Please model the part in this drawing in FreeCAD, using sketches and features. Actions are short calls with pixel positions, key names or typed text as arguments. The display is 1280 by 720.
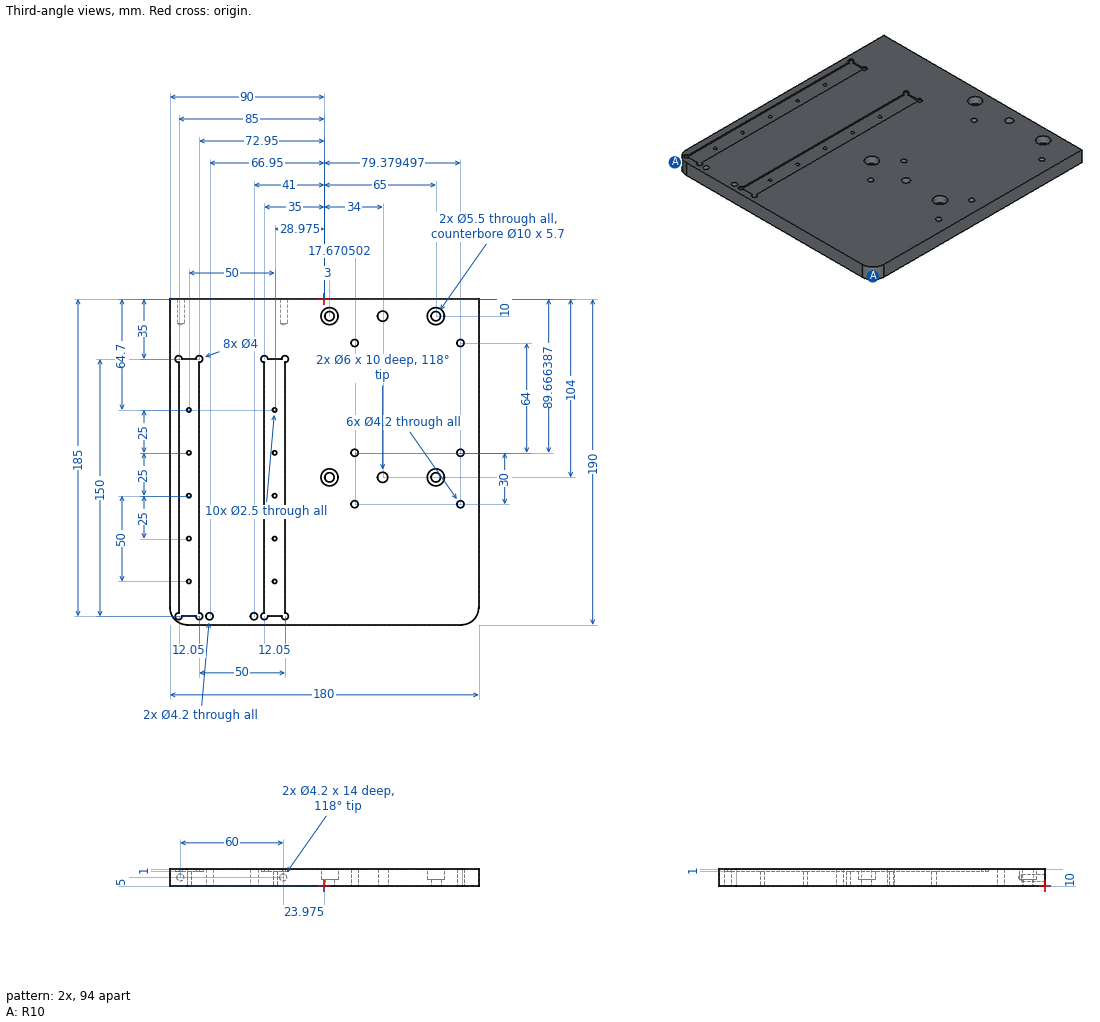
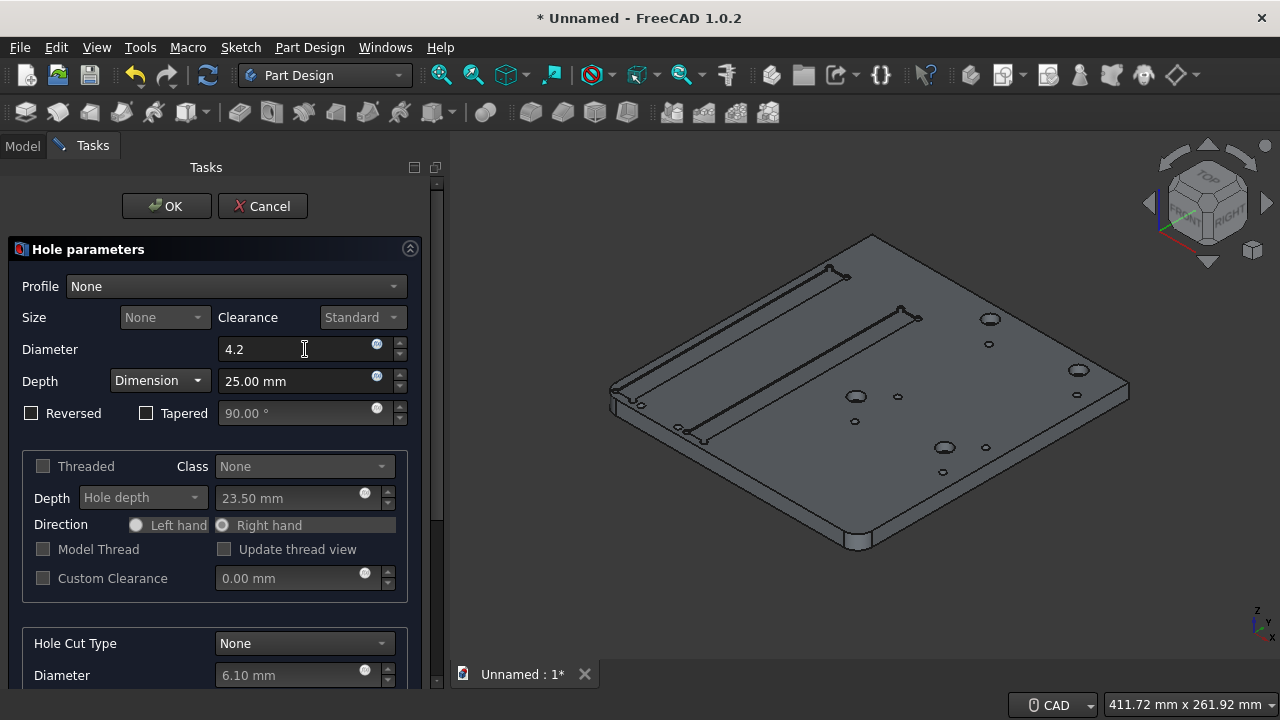
click(161, 380)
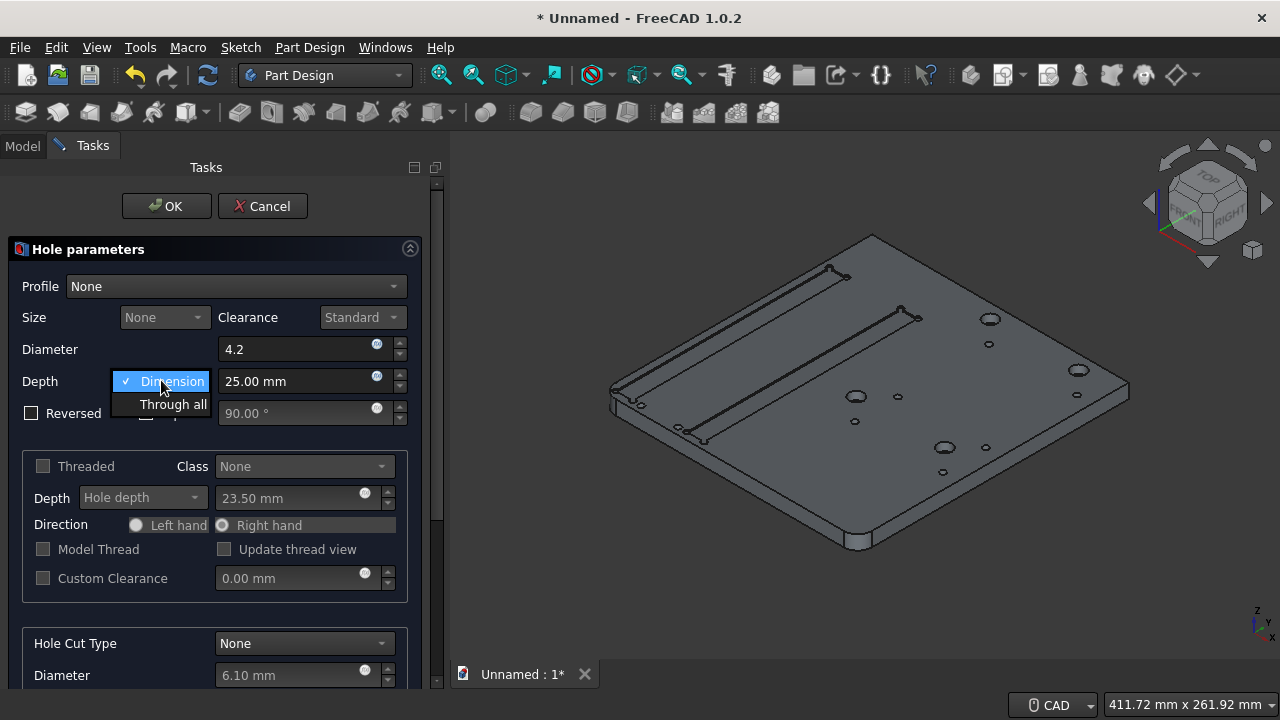
click(160, 404)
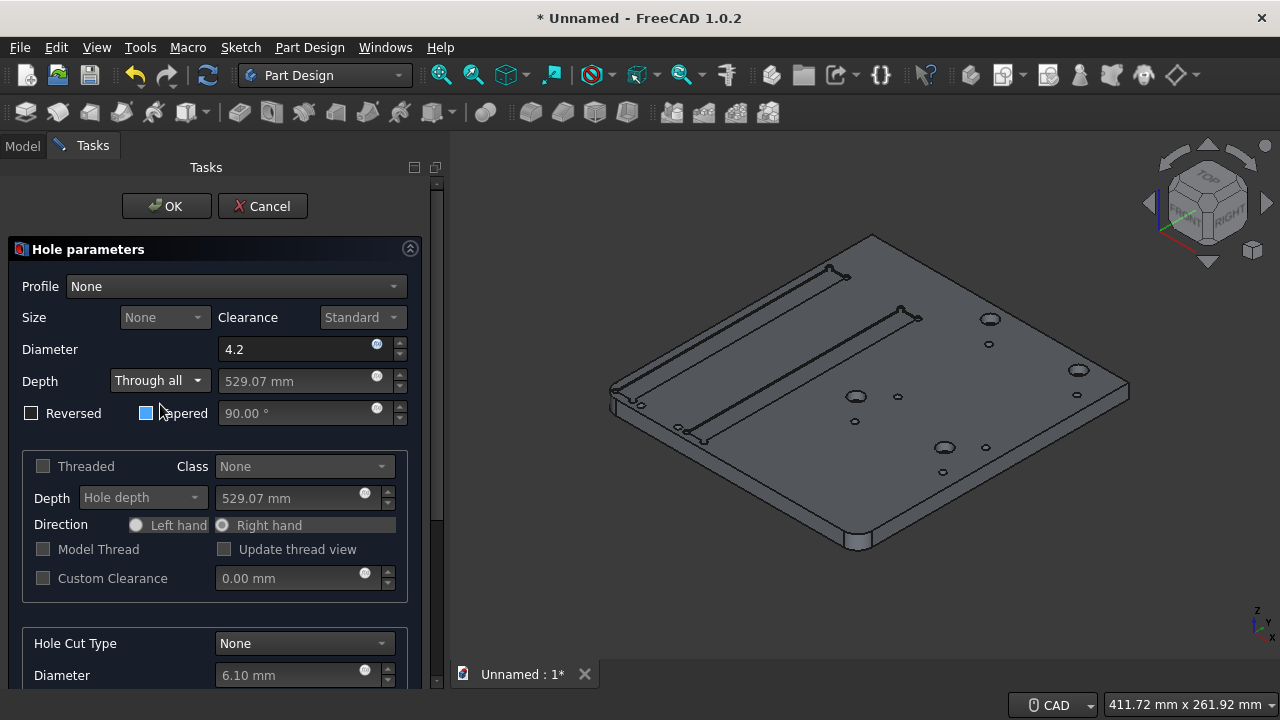
click(167, 206)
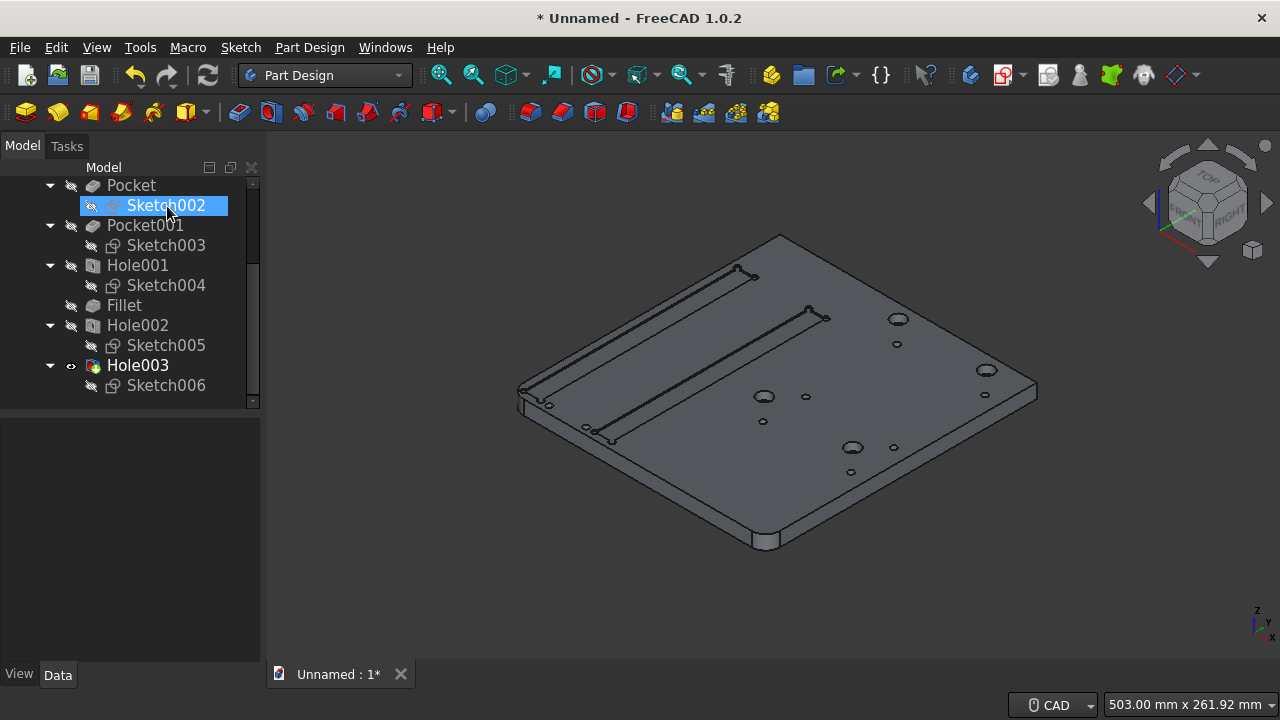
click(769, 473)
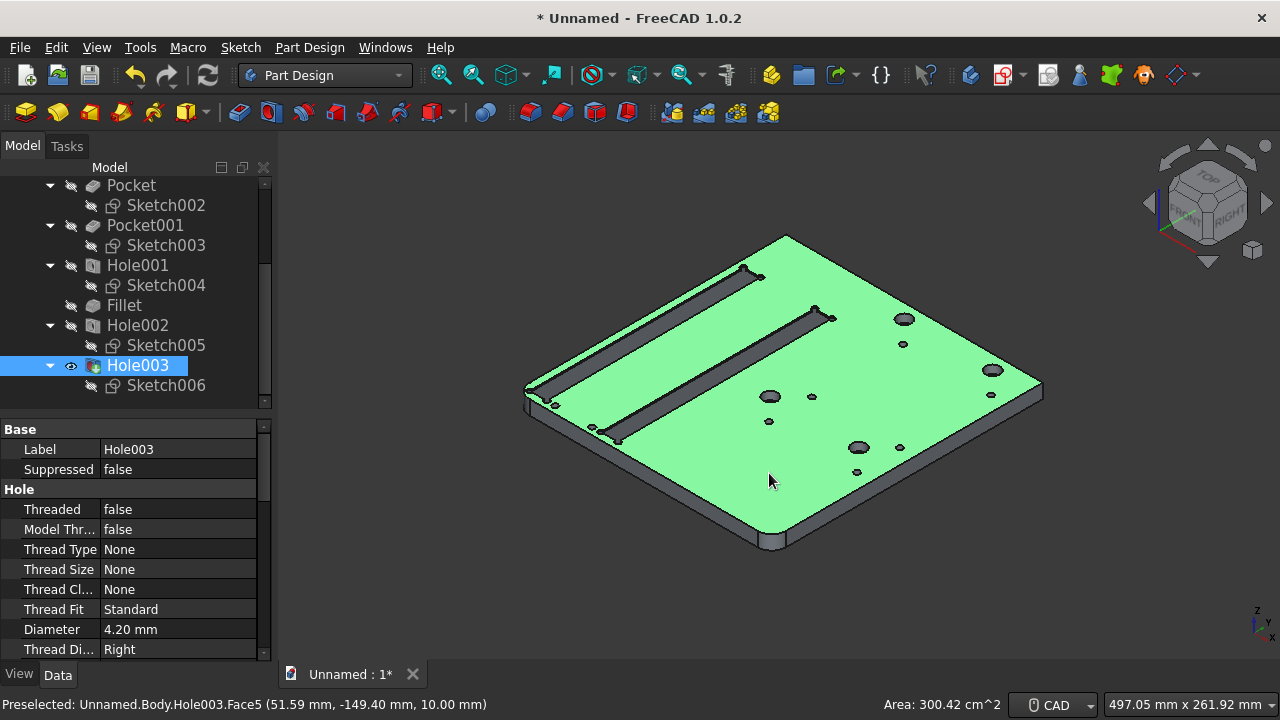
click(1004, 76)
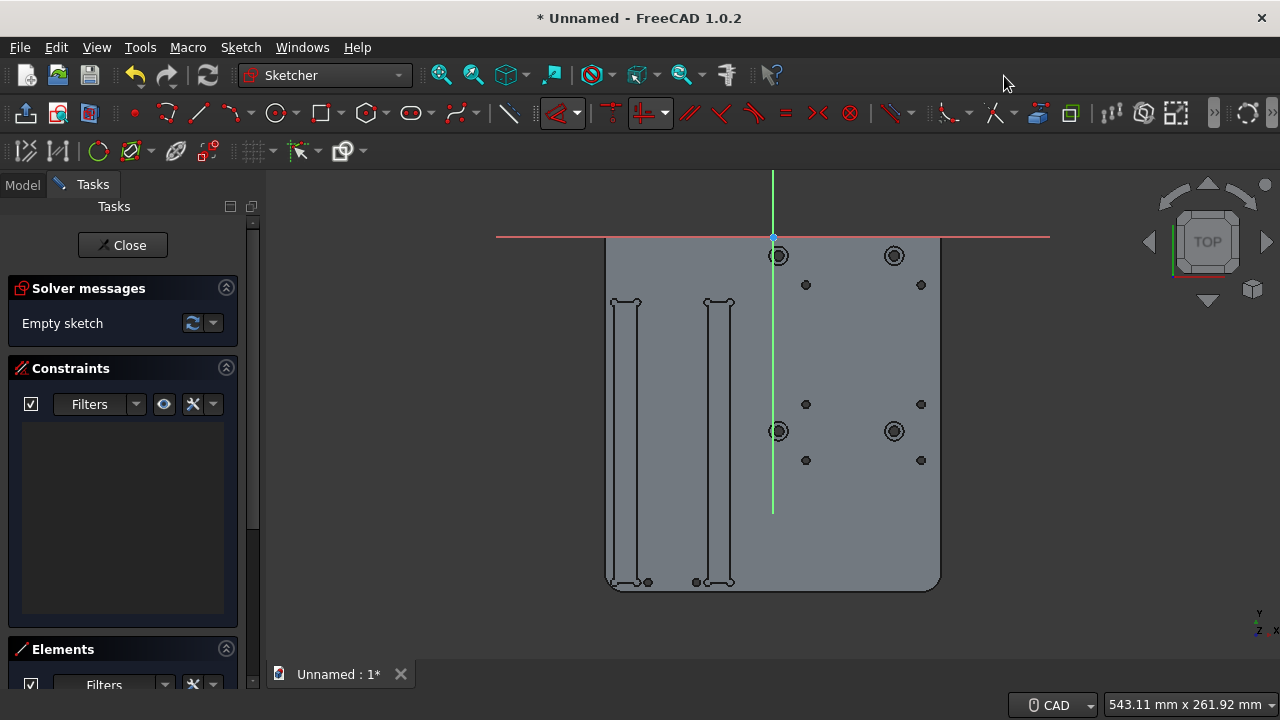
scroll(1017, 198, up, 2)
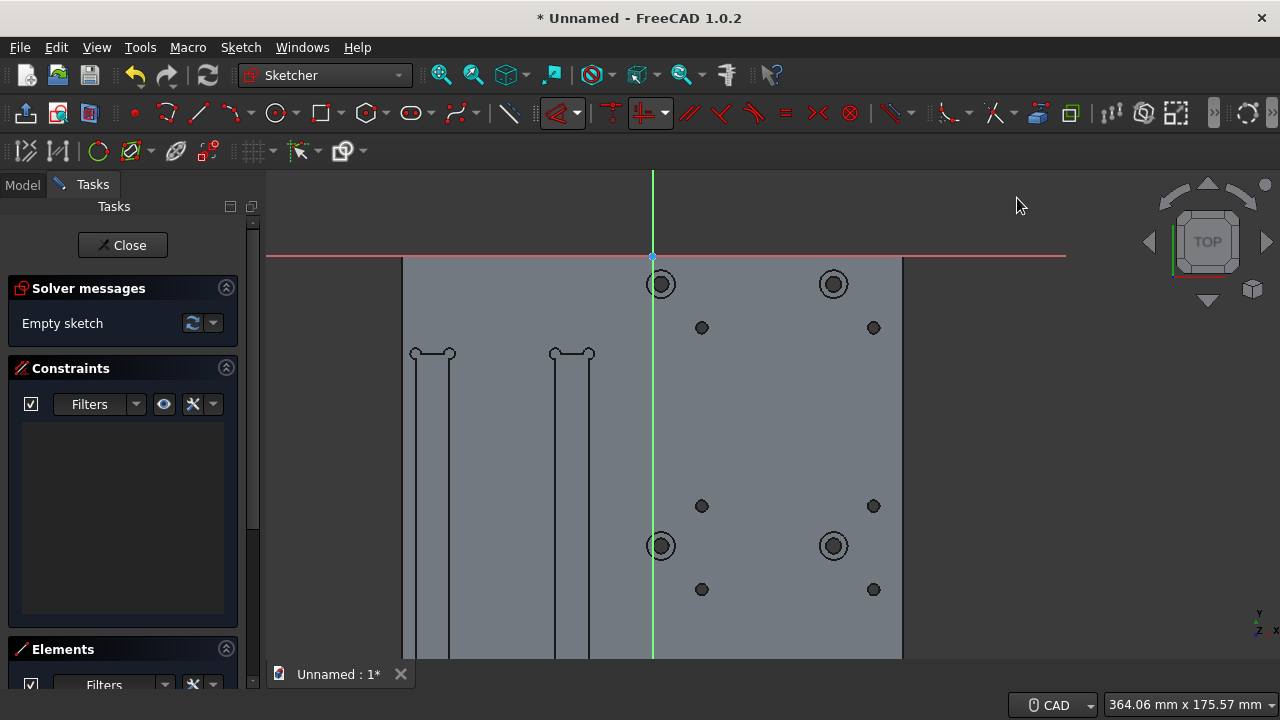
click(276, 114)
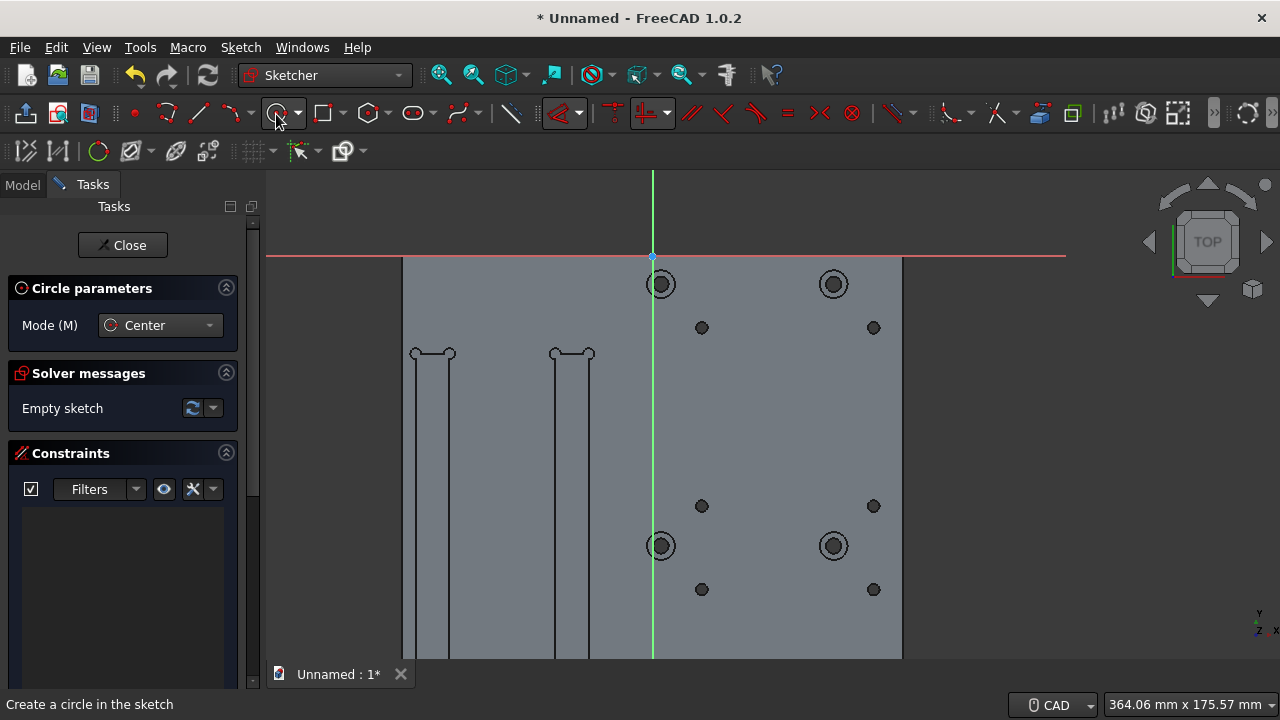
scroll(747, 546, up, 5)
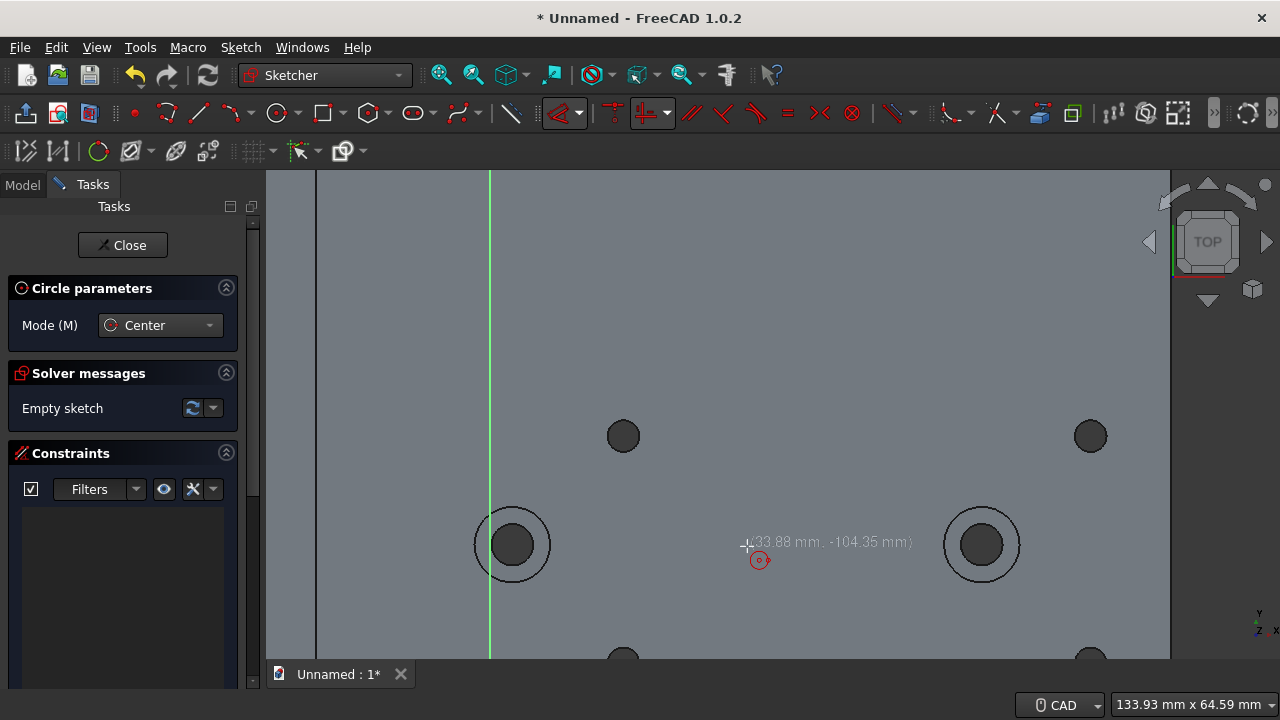
click(747, 545)
move(763, 529)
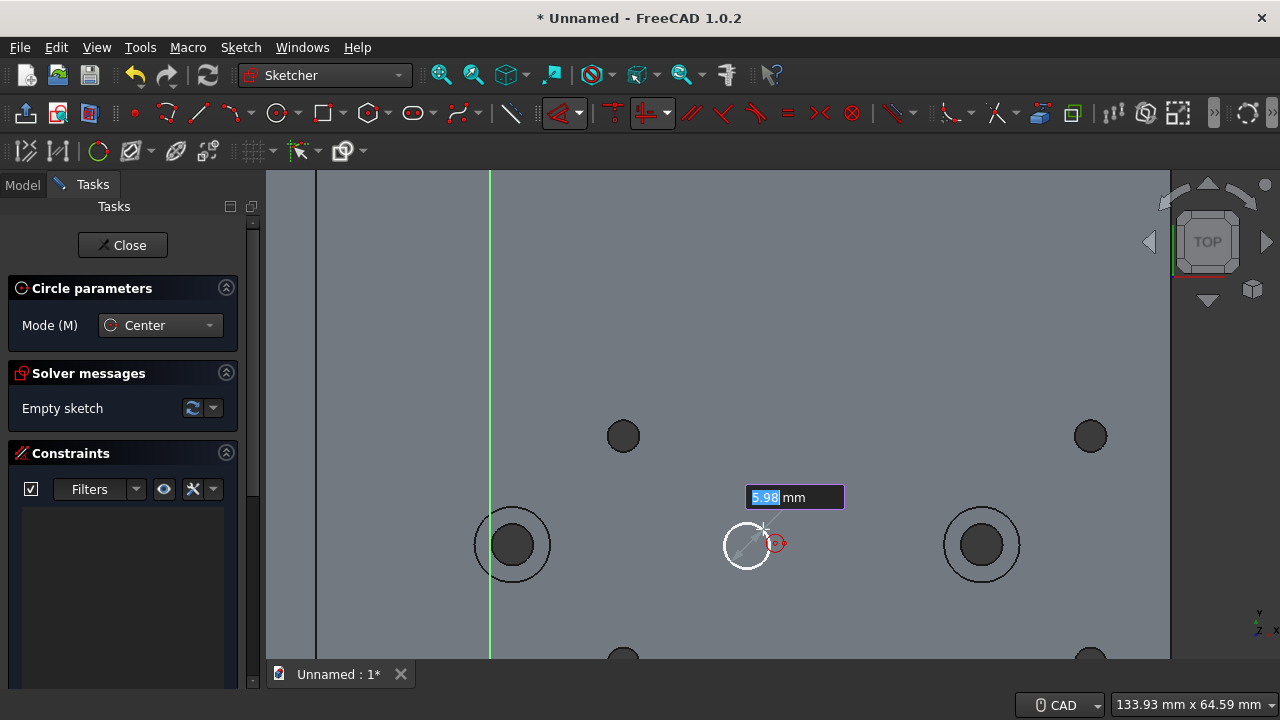
text(6)
key(Return)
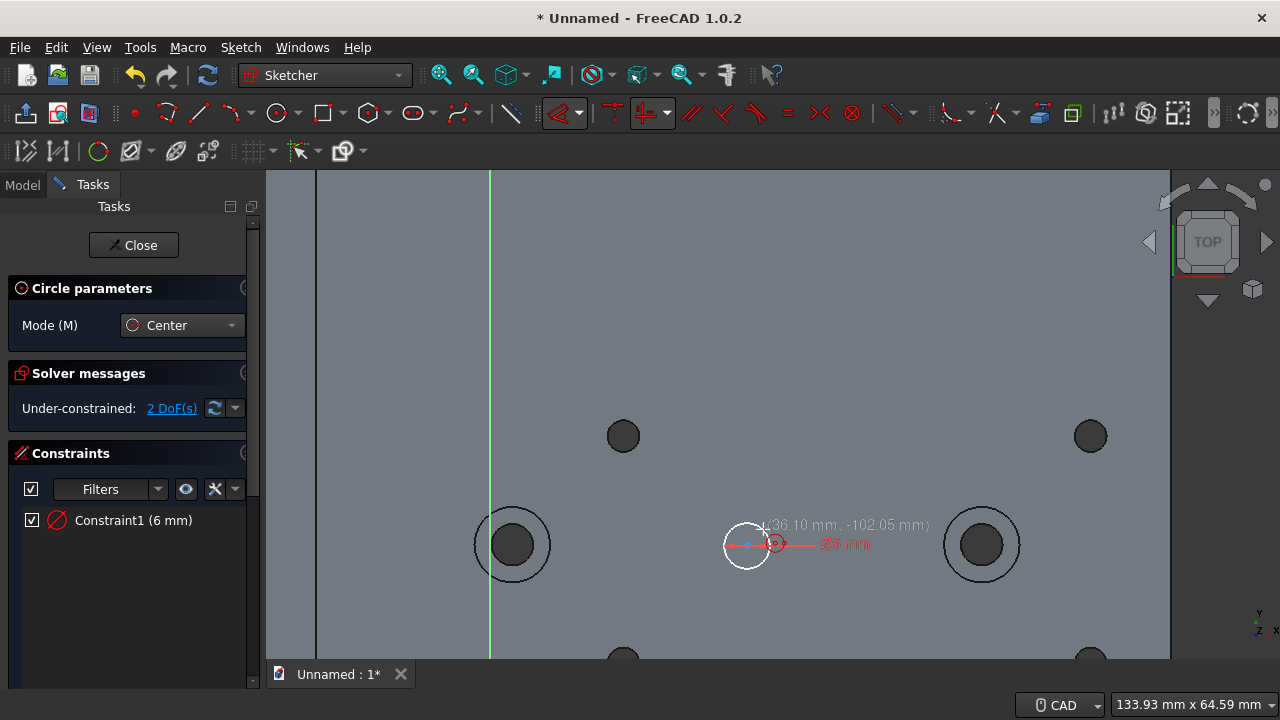
scroll(748, 561, down, 5)